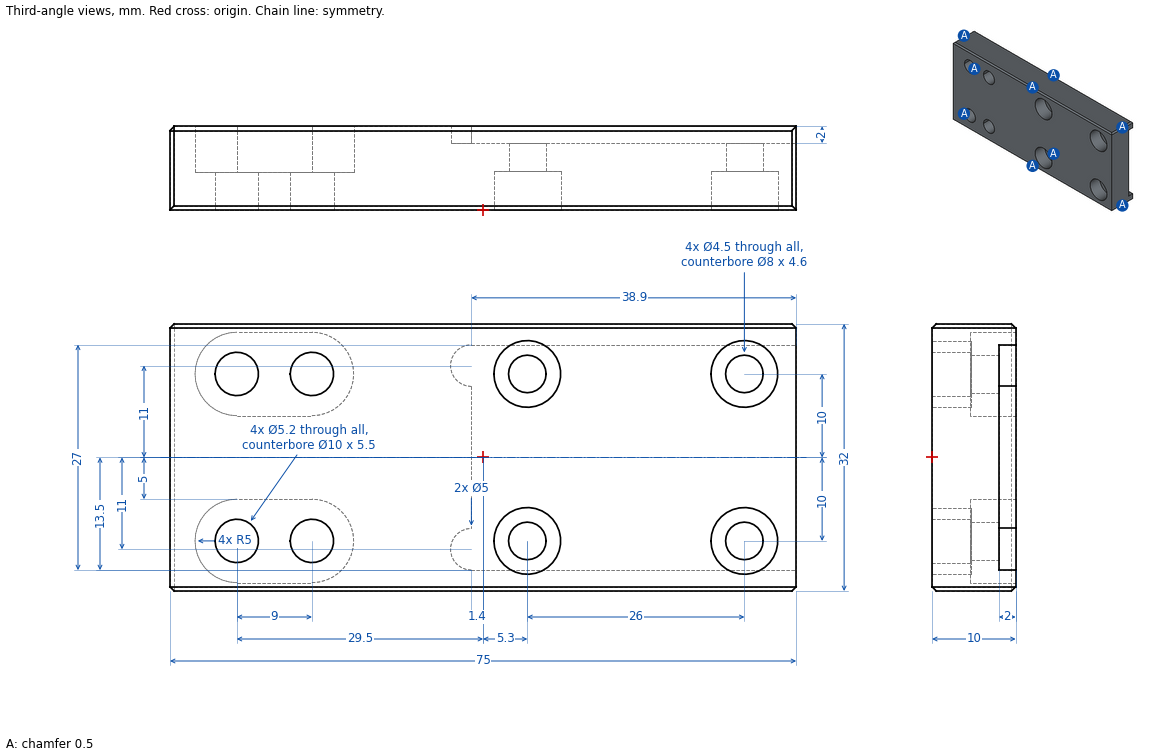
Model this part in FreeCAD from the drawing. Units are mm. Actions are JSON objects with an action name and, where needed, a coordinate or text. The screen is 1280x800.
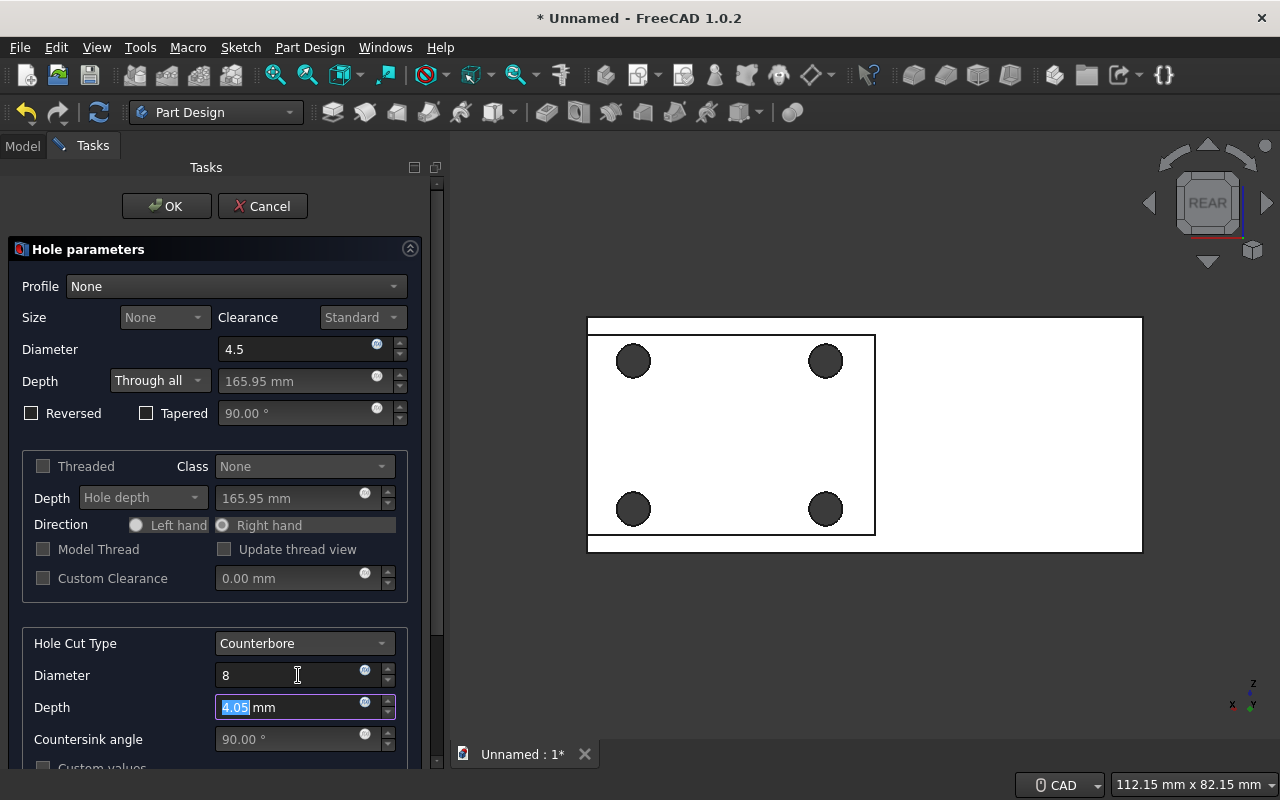
{"action": "type", "text": "4.6"}
{"action": "key", "text": "Tab"}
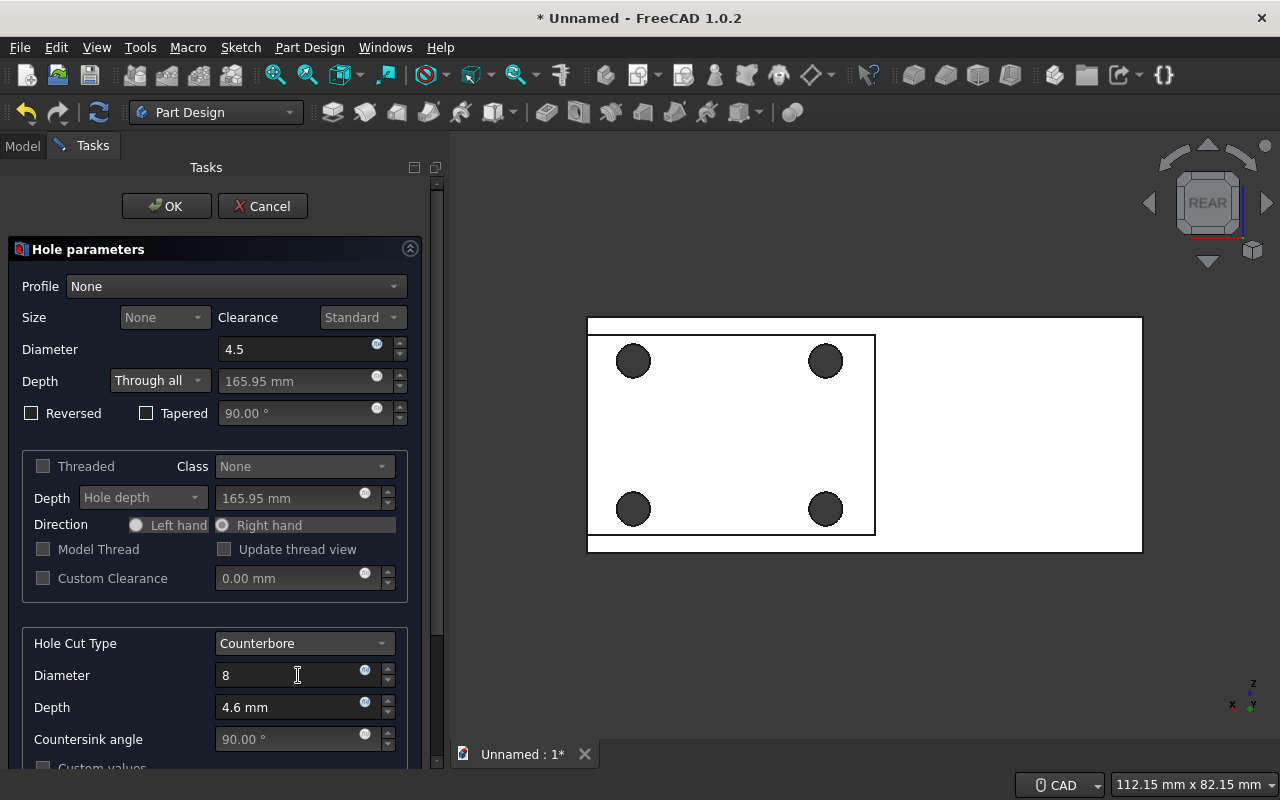
{"action": "left_click", "coordinate": [167, 206]}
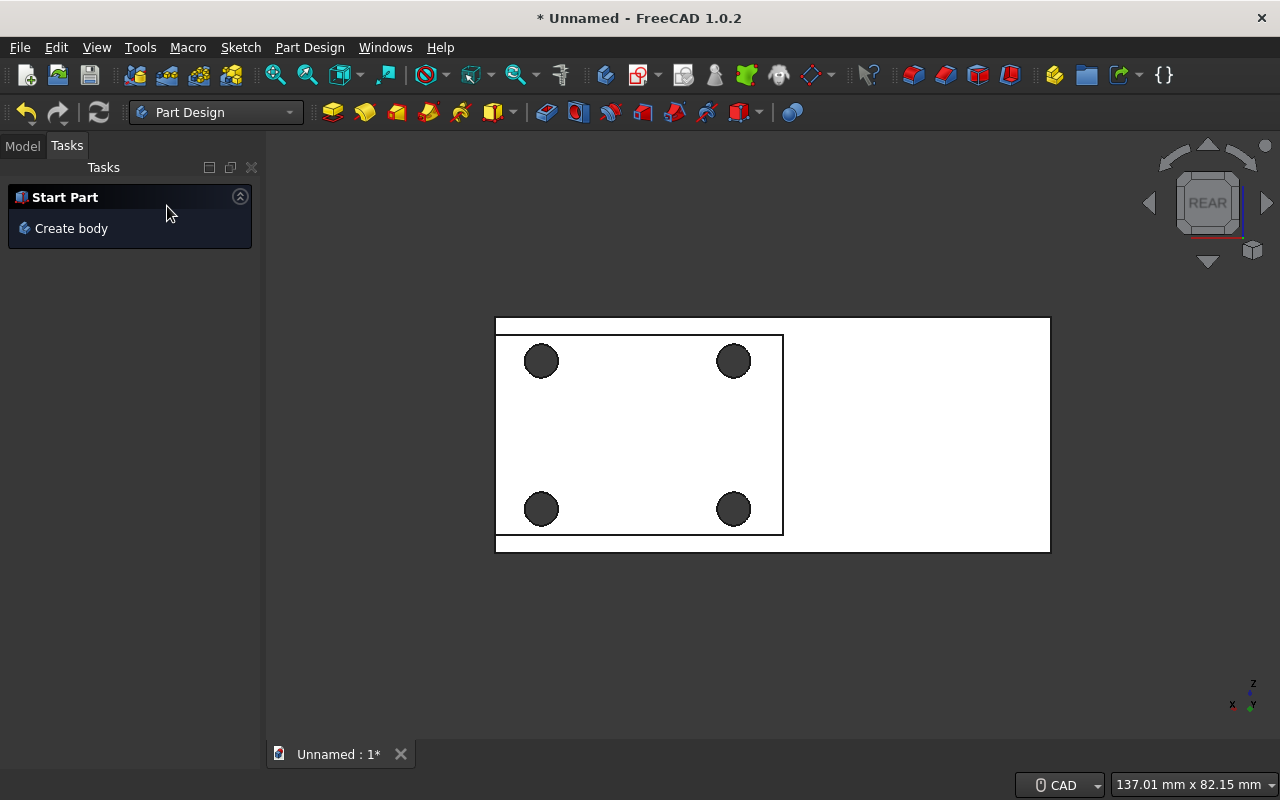
{"action": "left_click", "coordinate": [932, 434]}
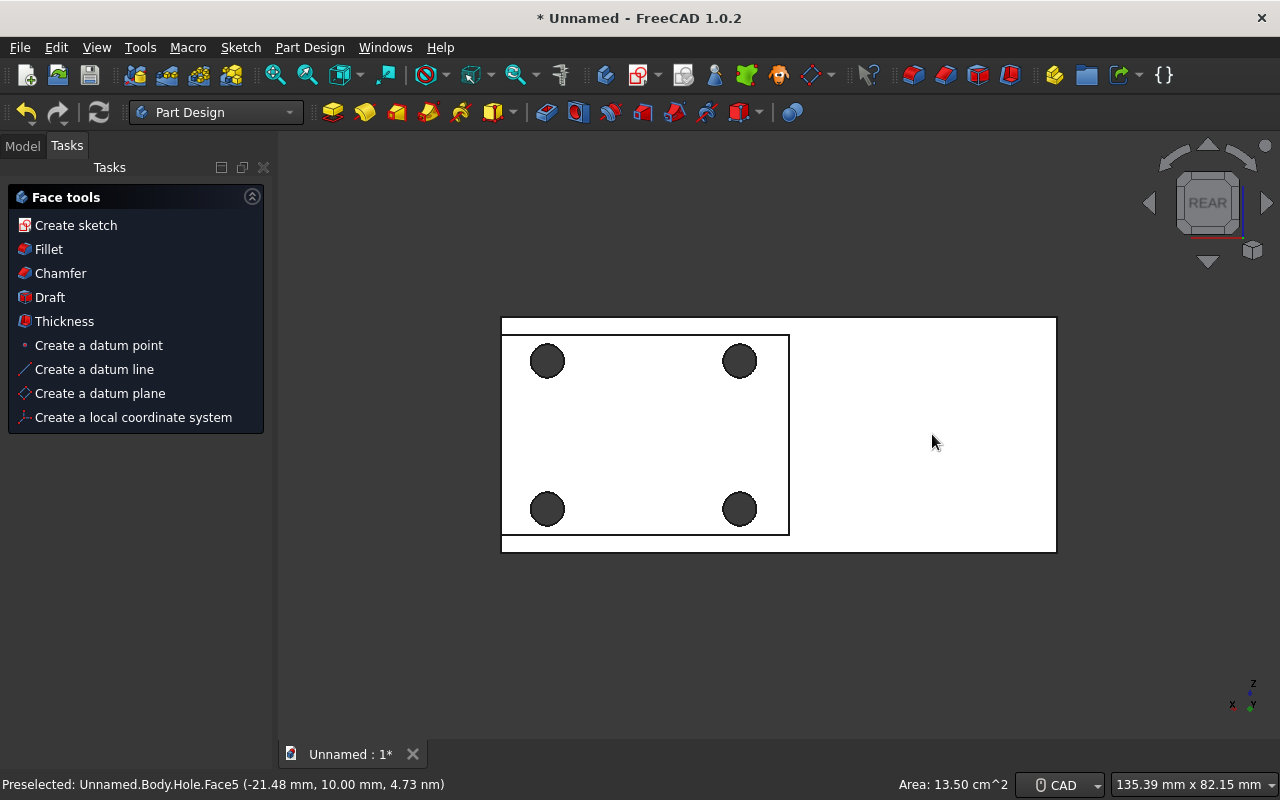
{"action": "left_click", "coordinate": [638, 76]}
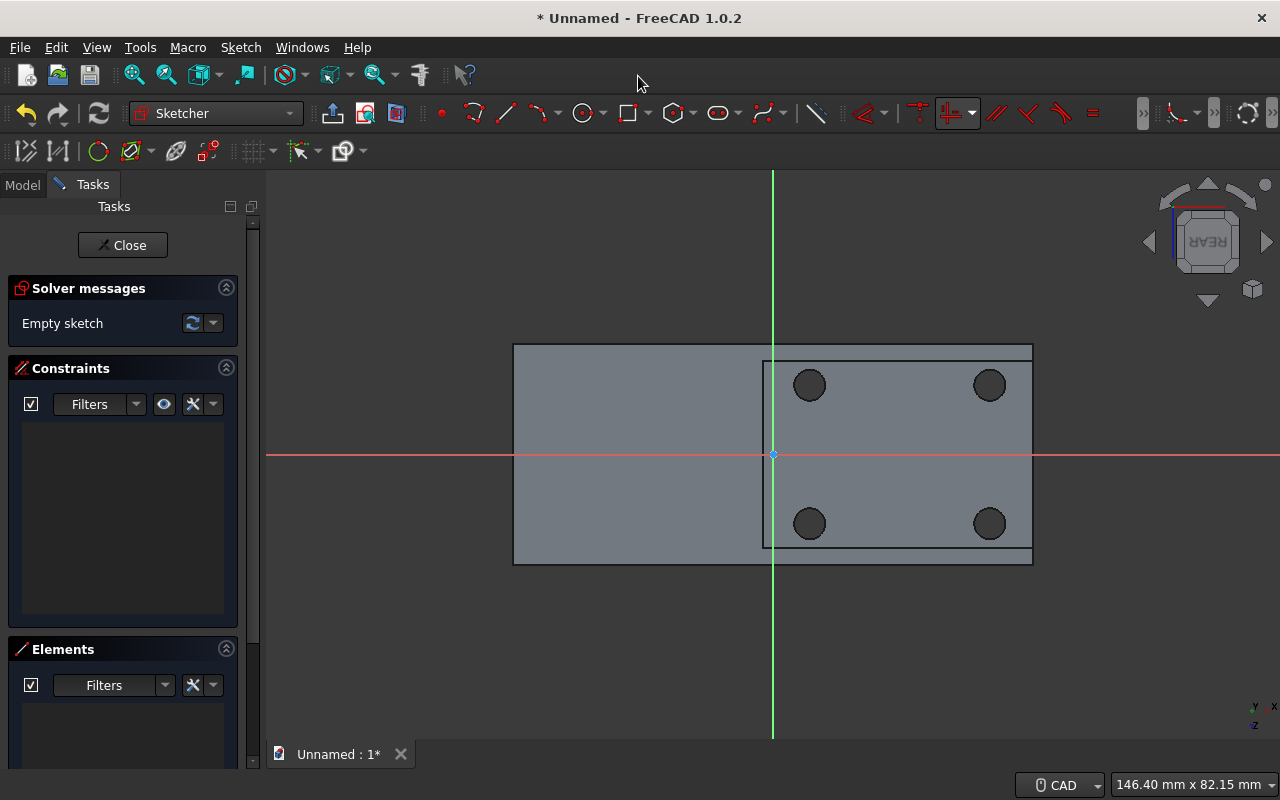
{"action": "scroll", "coordinate": [627, 454], "scroll_direction": "up", "scroll_amount": 4}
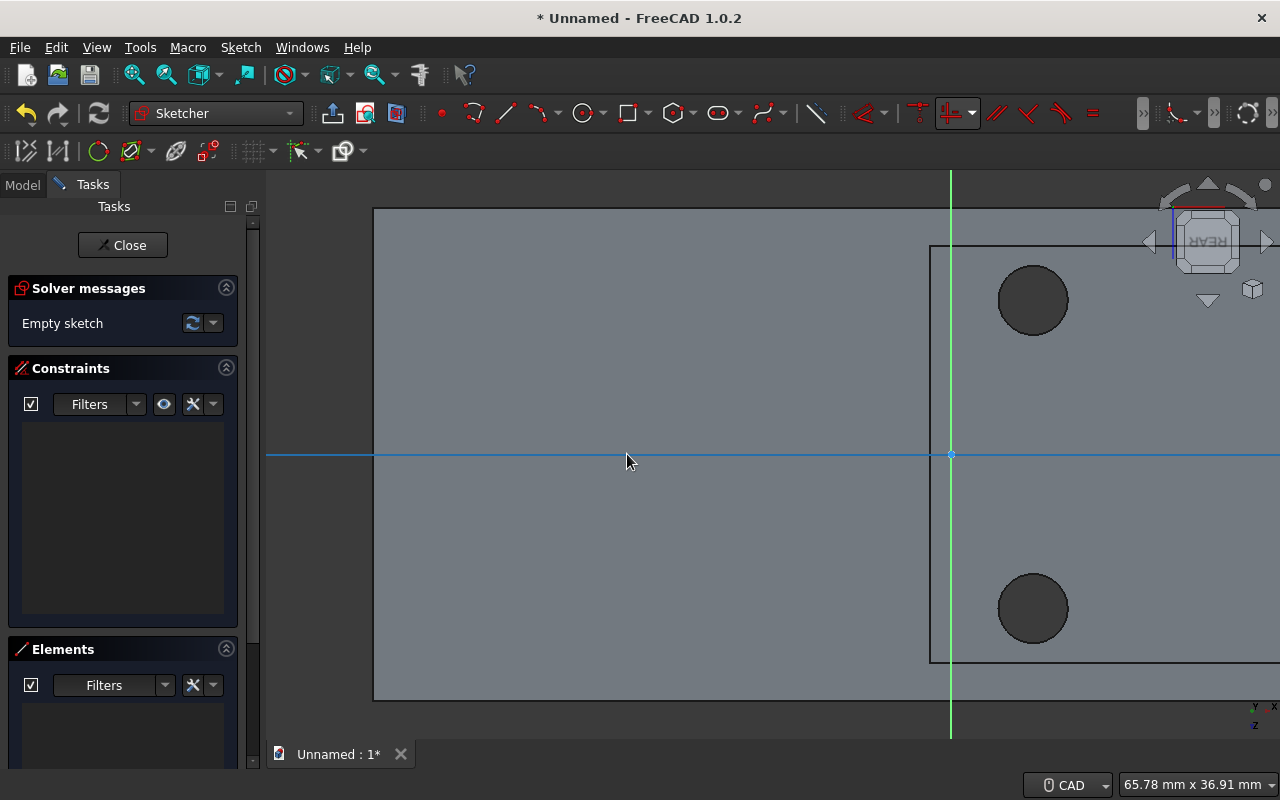
{"action": "left_click", "coordinate": [584, 114]}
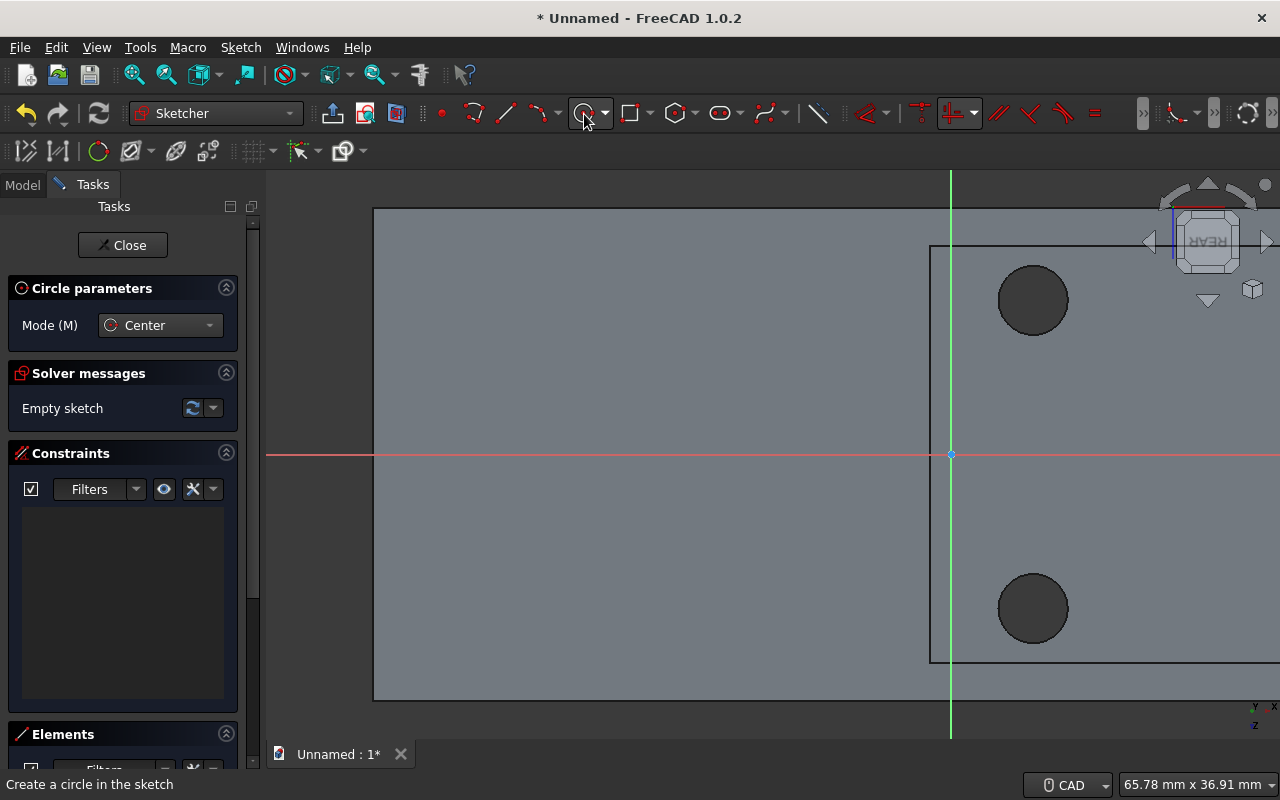
{"action": "left_click", "coordinate": [497, 300]}
{"action": "left_click", "coordinate": [525, 272]}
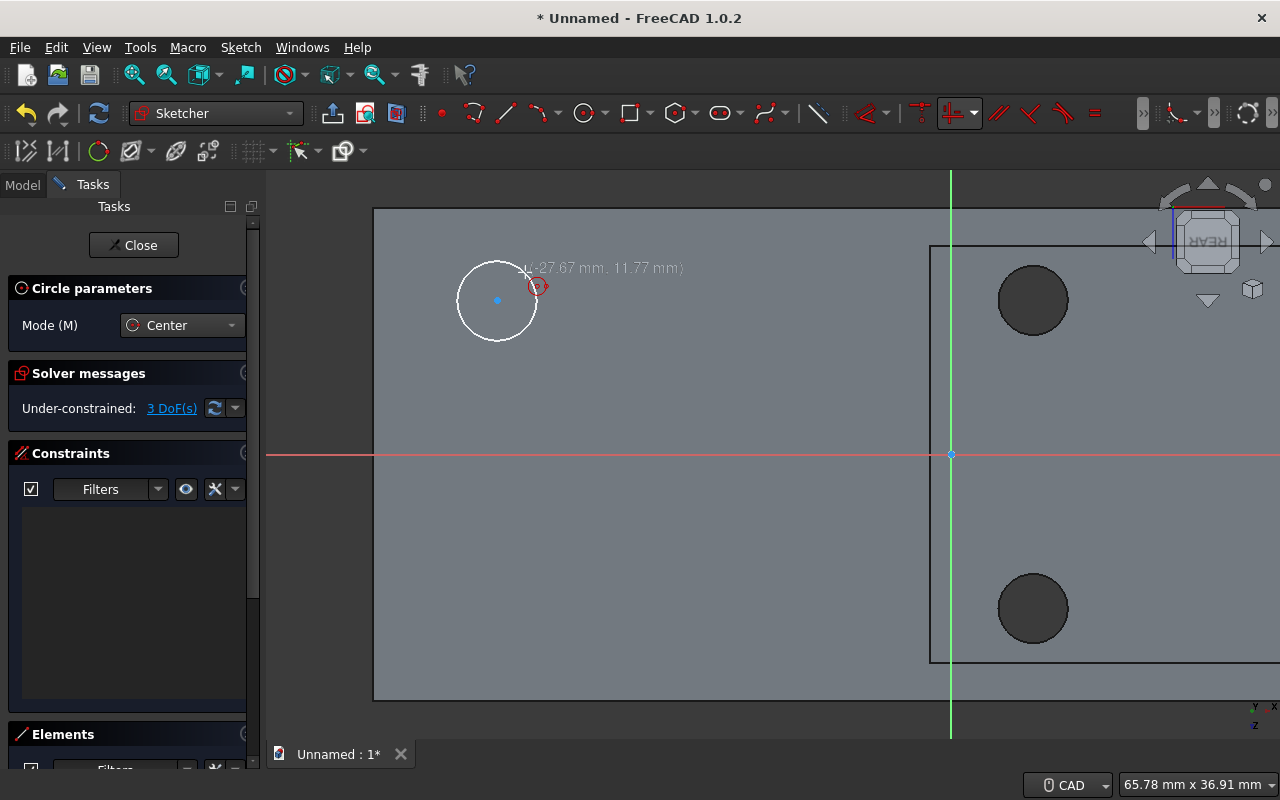
{"action": "left_click", "coordinate": [635, 300]}
{"action": "left_click", "coordinate": [664, 272]}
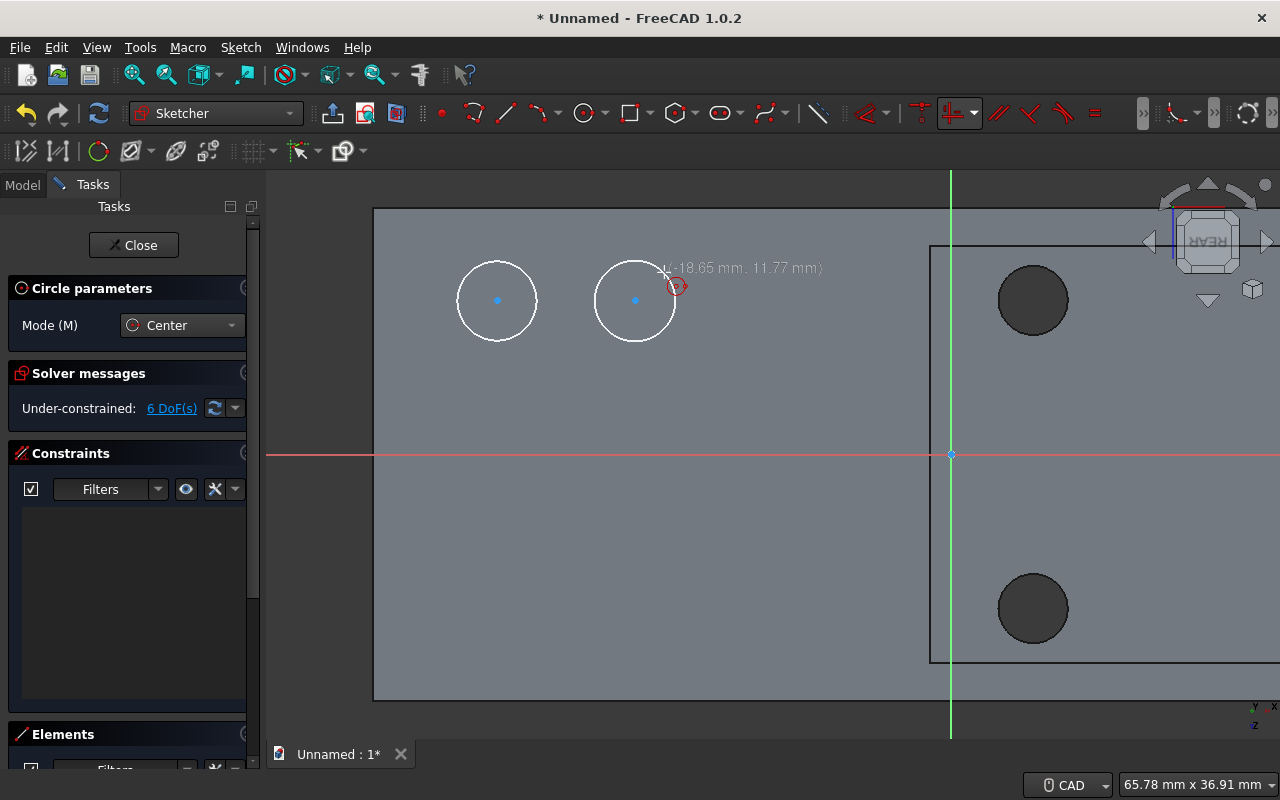
{"action": "left_click", "coordinate": [635, 609]}
{"action": "left_click", "coordinate": [664, 580]}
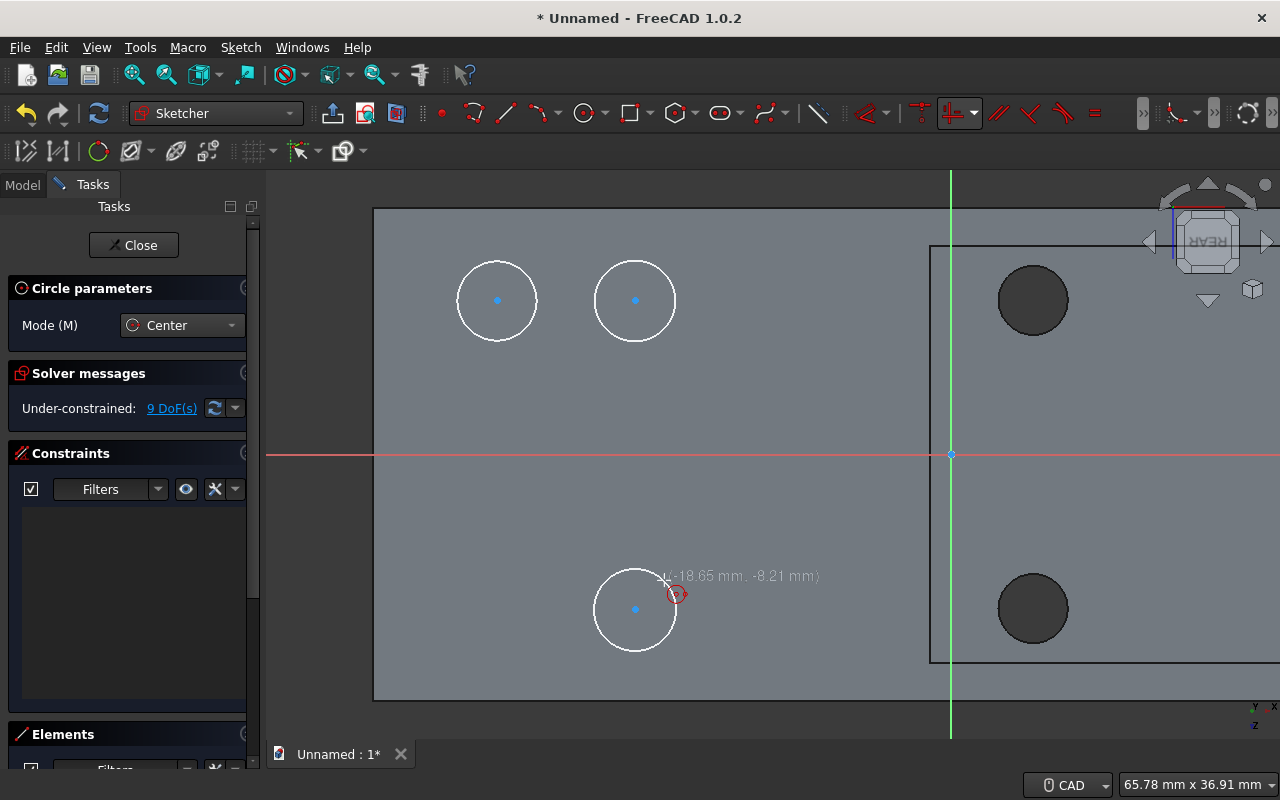
{"action": "left_click", "coordinate": [497, 609]}
{"action": "left_click", "coordinate": [525, 580]}
{"action": "key", "text": "Escape"}